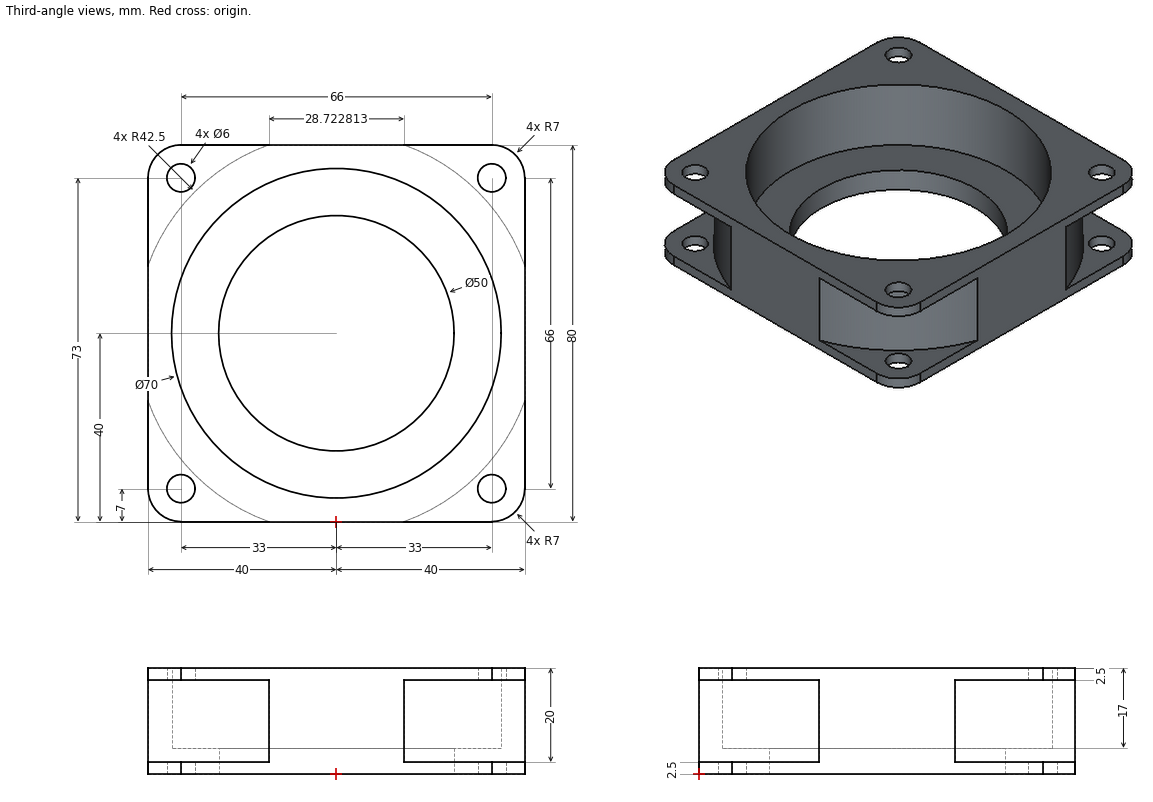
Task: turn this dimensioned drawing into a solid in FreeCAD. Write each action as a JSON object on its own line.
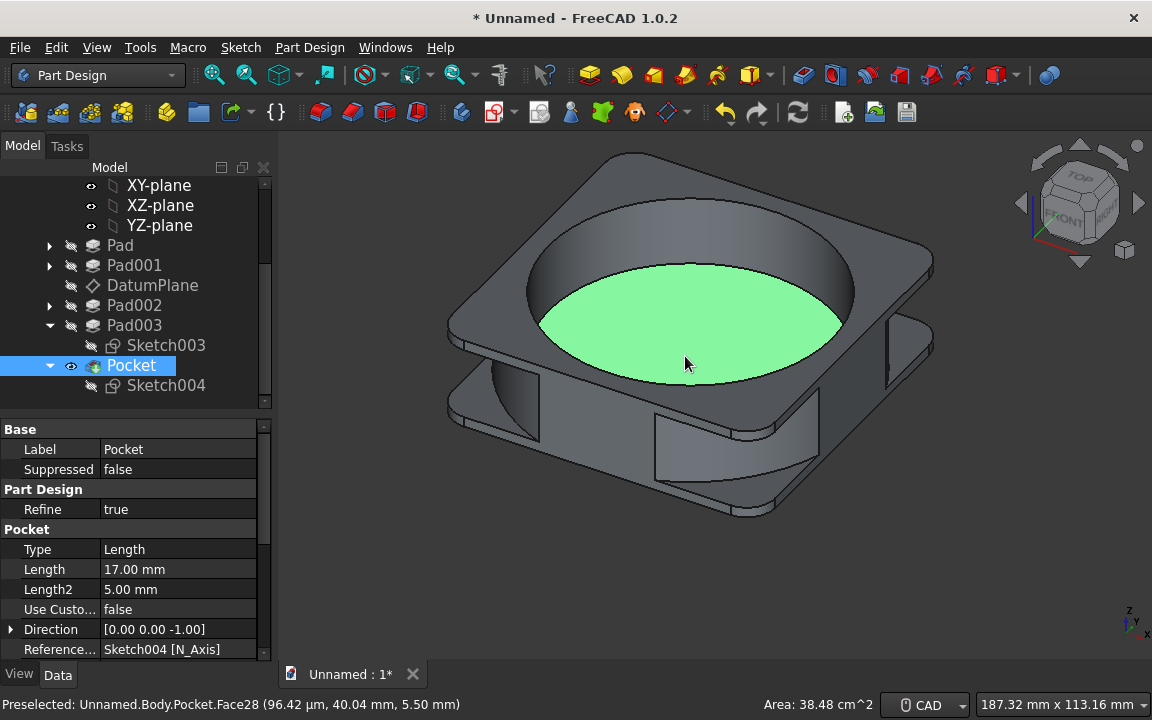
{"action": "left_click", "coordinate": [494, 112]}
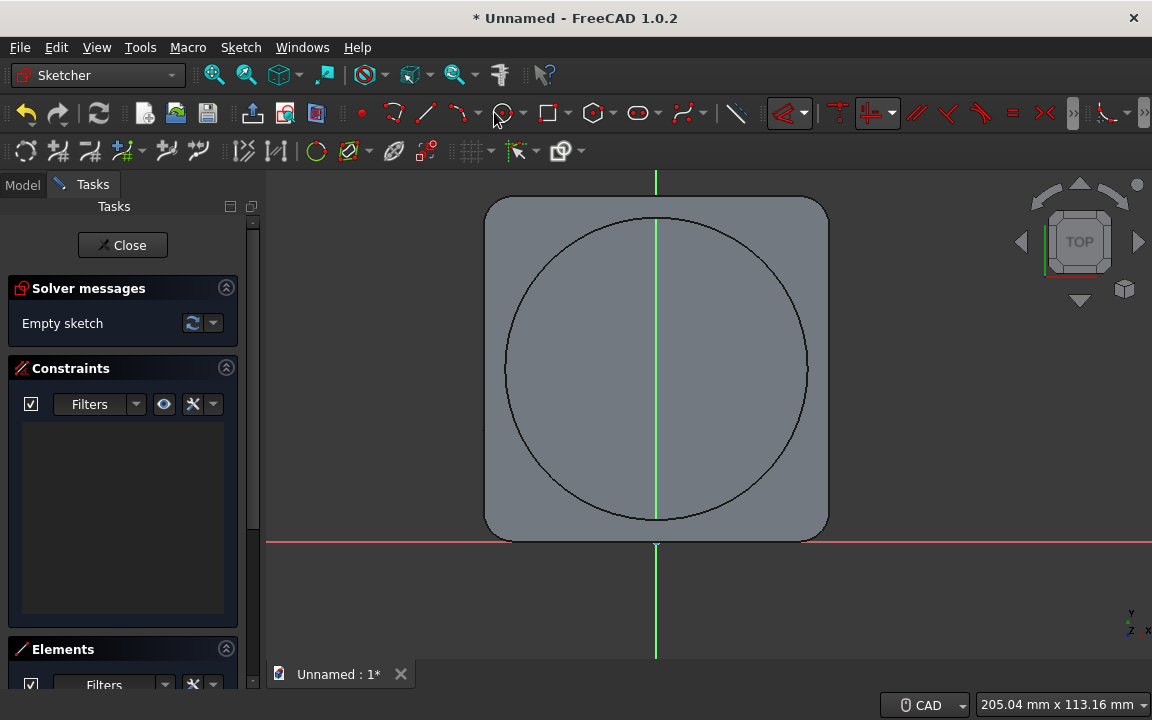
{"action": "key", "text": "g c"}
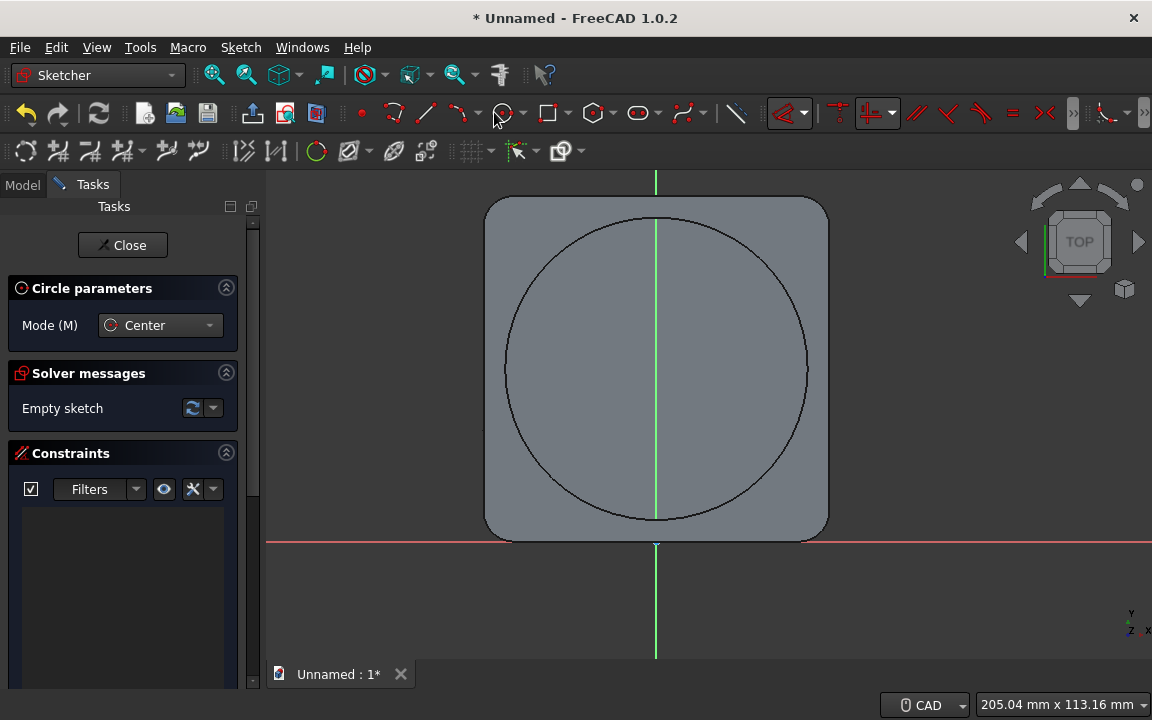
{"action": "left_click", "coordinate": [656, 369]}
{"action": "mouse_move", "coordinate": [733, 292]}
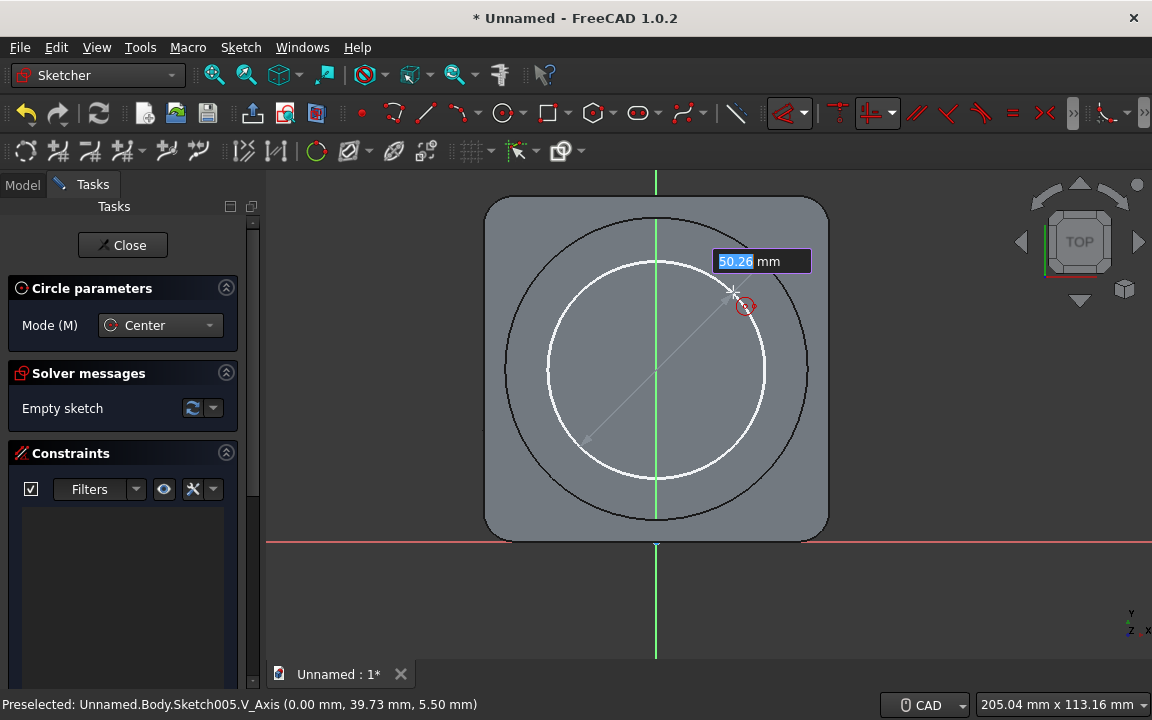
{"action": "type", "text": "50"}
{"action": "key", "text": "Return"}
{"action": "key", "text": "Escape"}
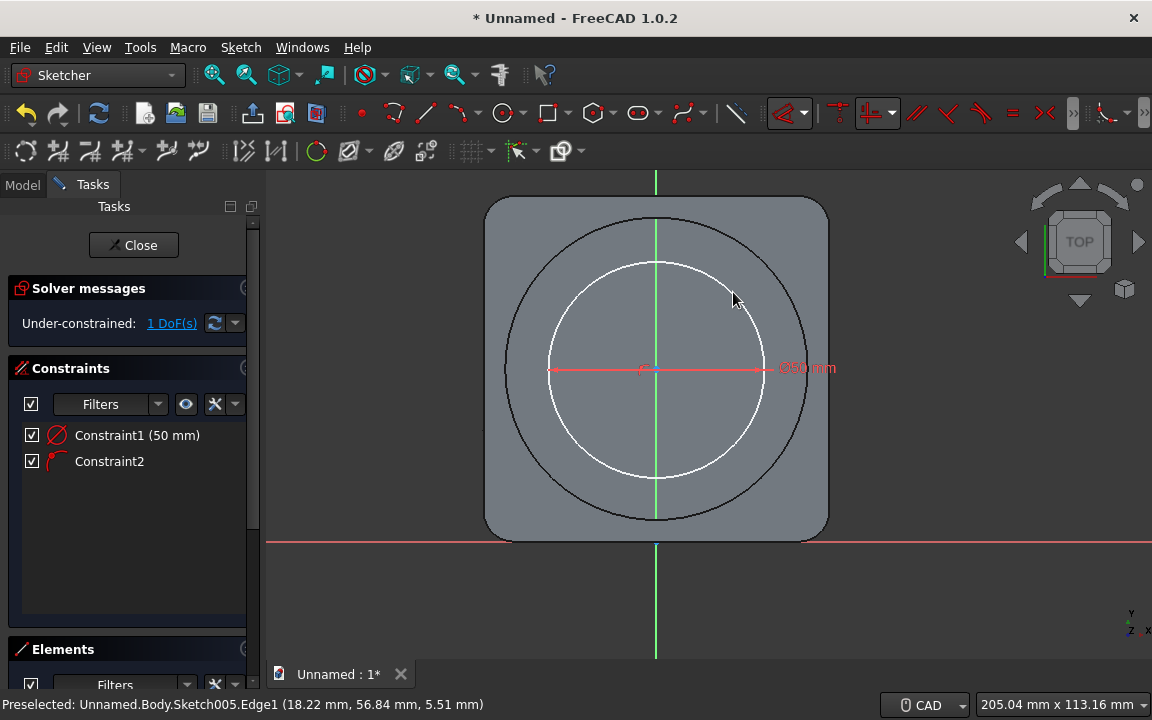
{"action": "left_click", "coordinate": [784, 114]}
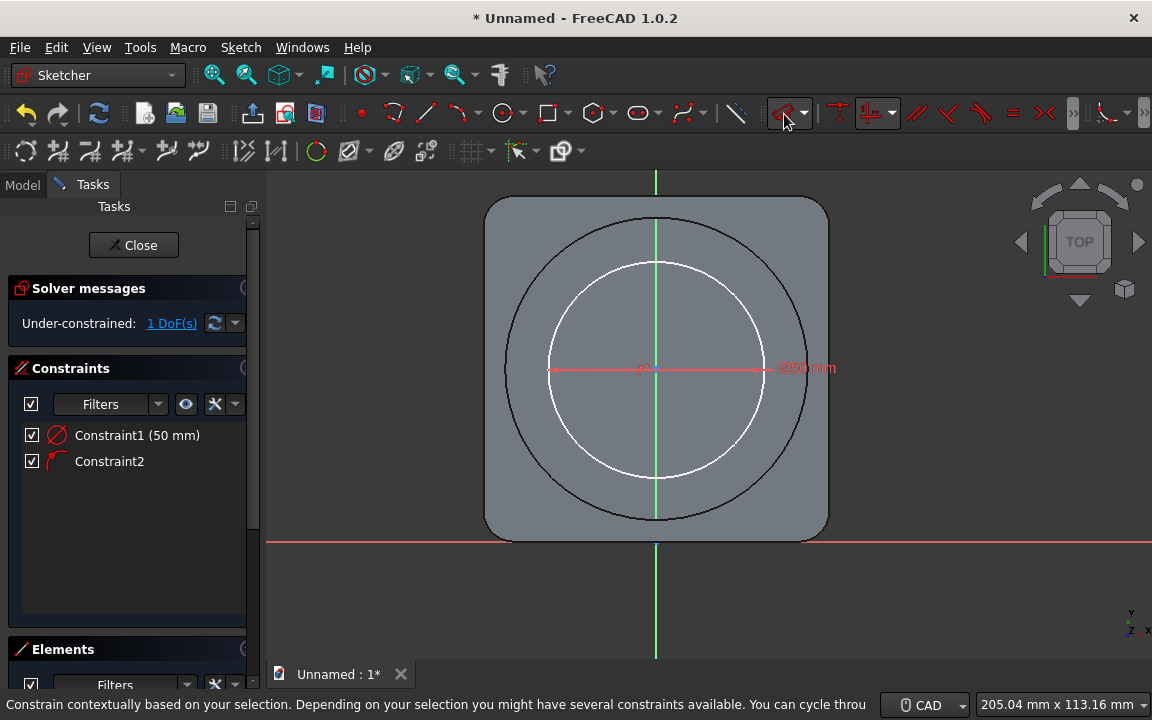
{"action": "left_click", "coordinate": [656, 370]}
{"action": "left_click", "coordinate": [690, 456]}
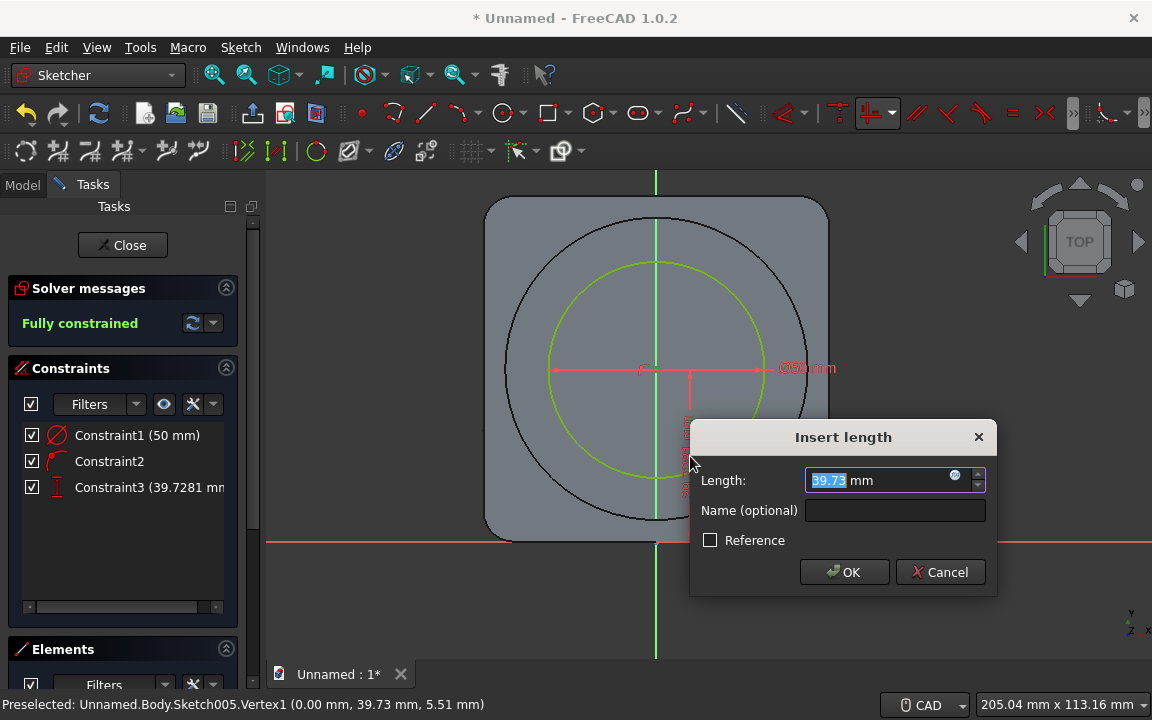
{"action": "type", "text": "40"}
{"action": "key", "text": "Return"}
{"action": "key", "text": "Escape"}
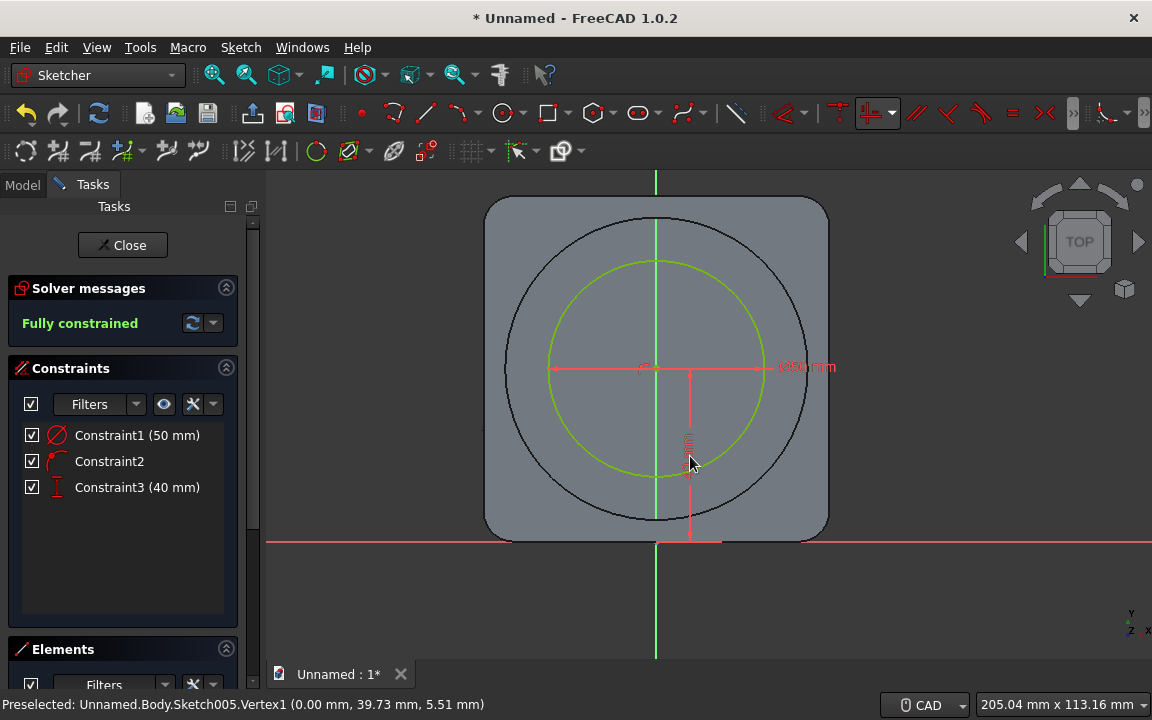
{"action": "left_click", "coordinate": [123, 245]}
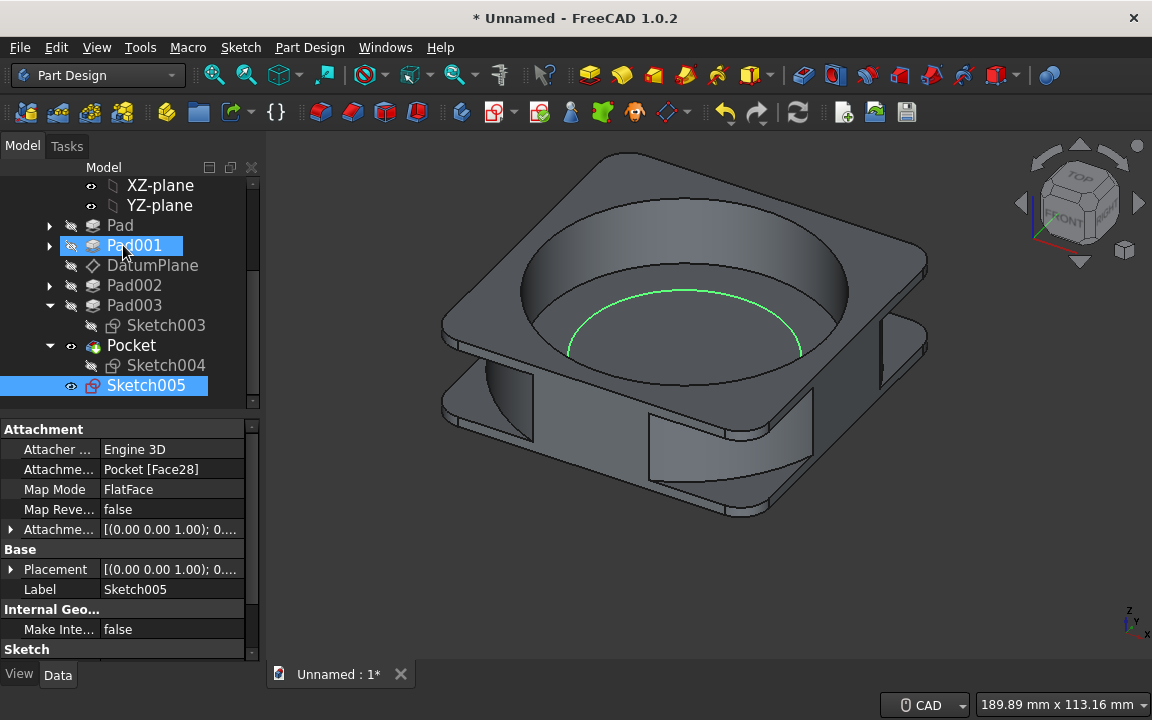
{"action": "left_click", "coordinate": [804, 76]}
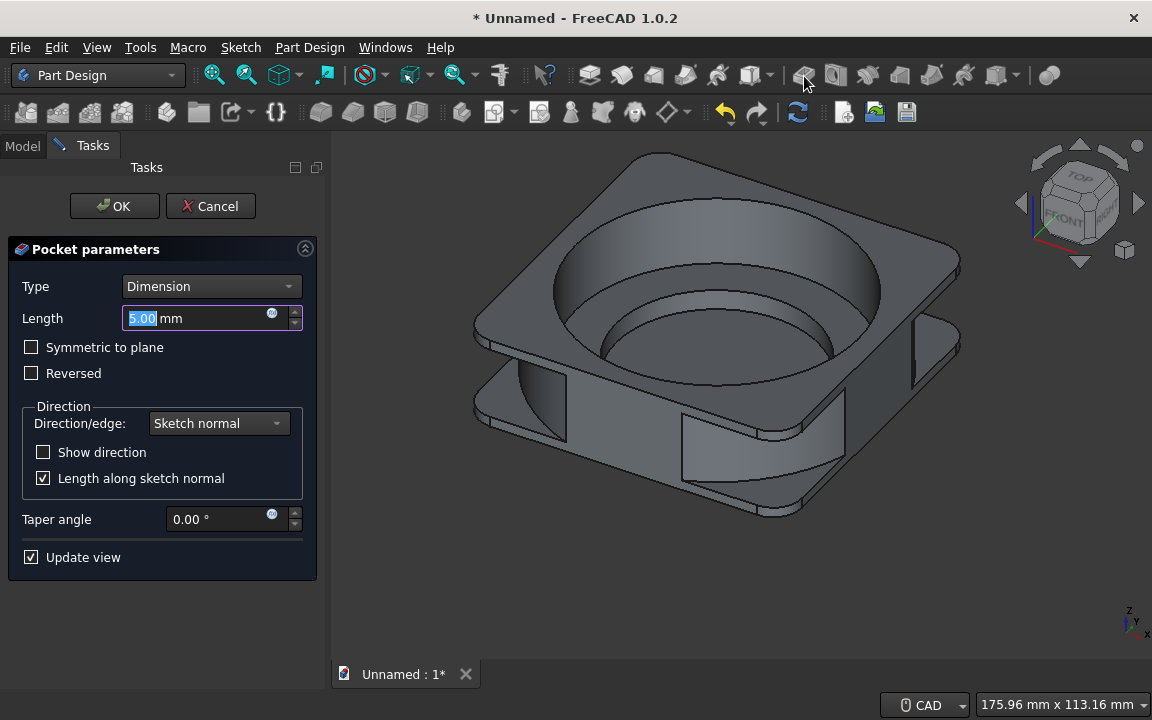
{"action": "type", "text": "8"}
{"action": "key", "text": "Tab"}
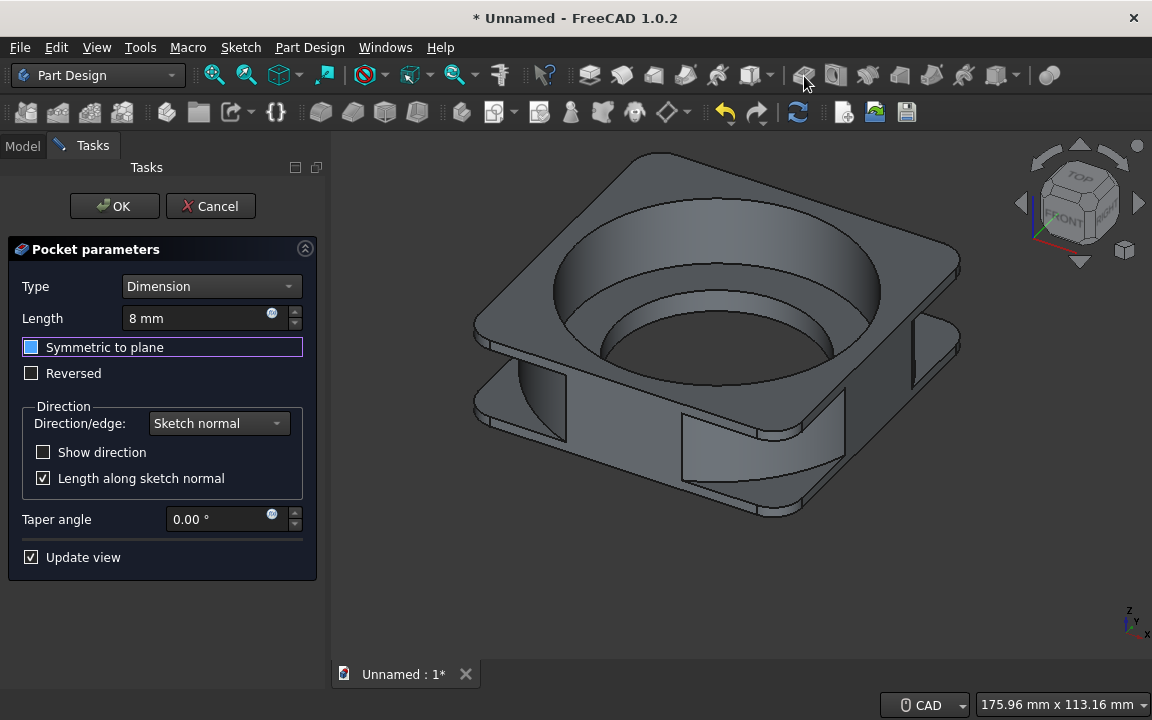
{"action": "left_click", "coordinate": [115, 206]}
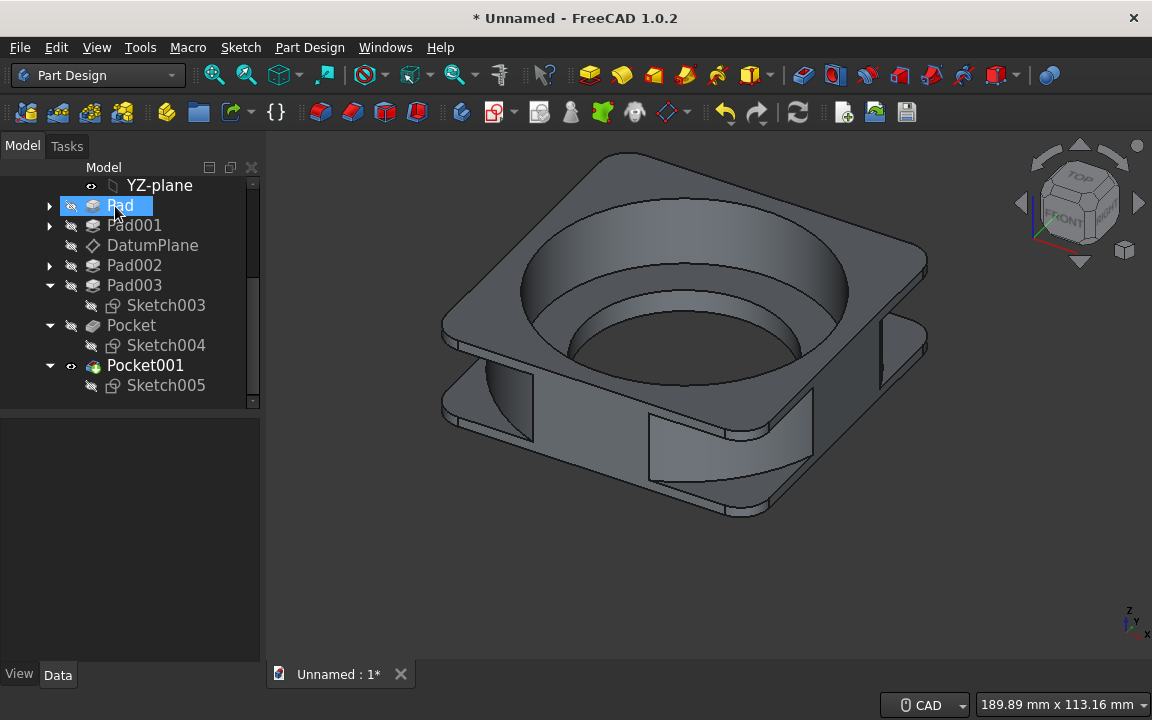
{"action": "left_click", "coordinate": [697, 401]}